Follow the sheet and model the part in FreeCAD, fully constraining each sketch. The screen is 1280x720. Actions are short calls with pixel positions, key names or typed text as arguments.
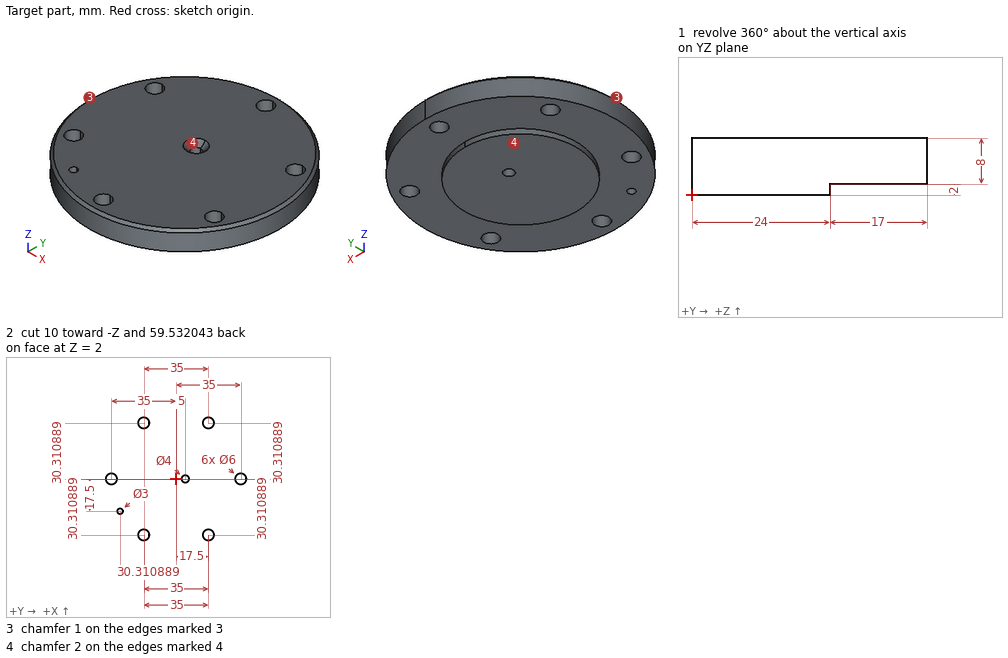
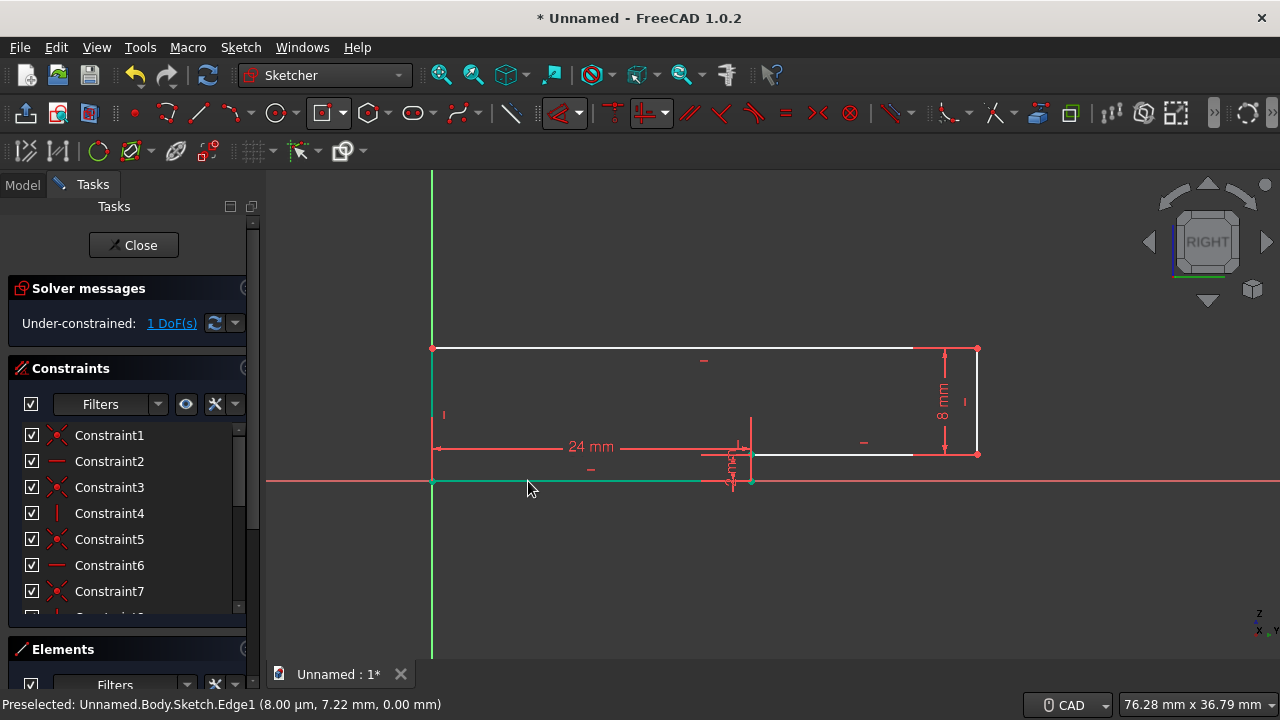
click(819, 455)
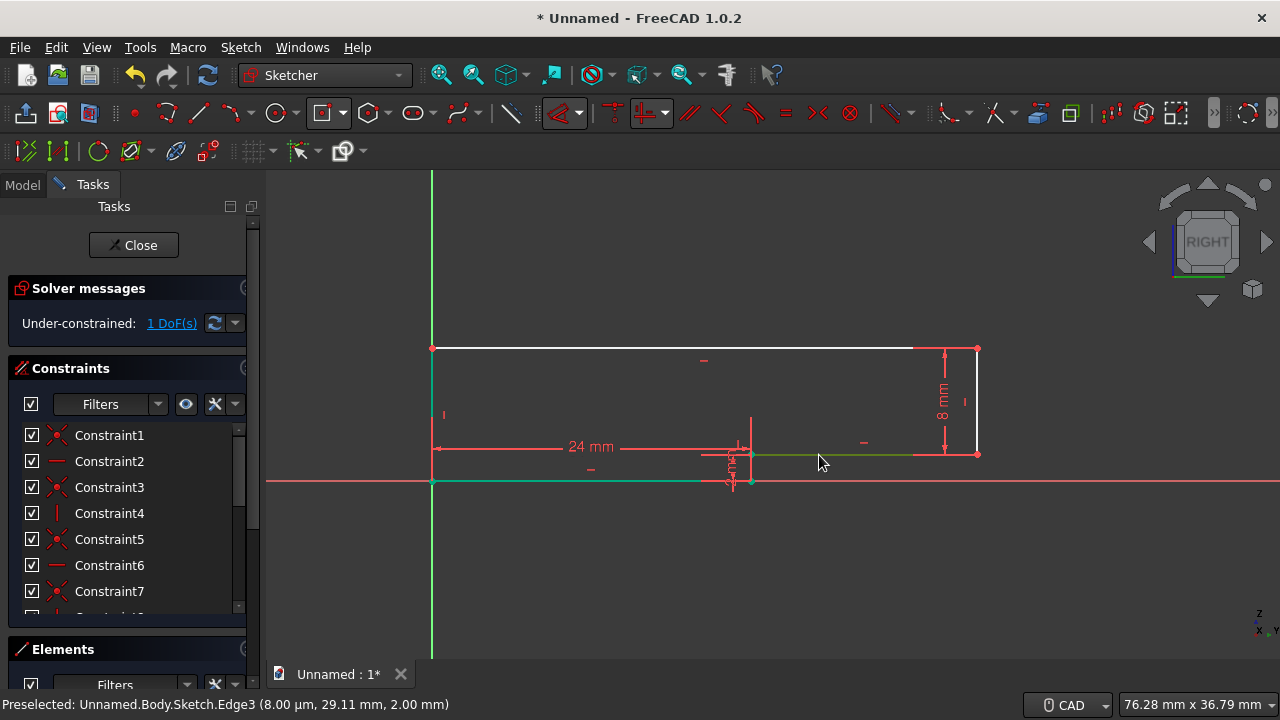
key(l)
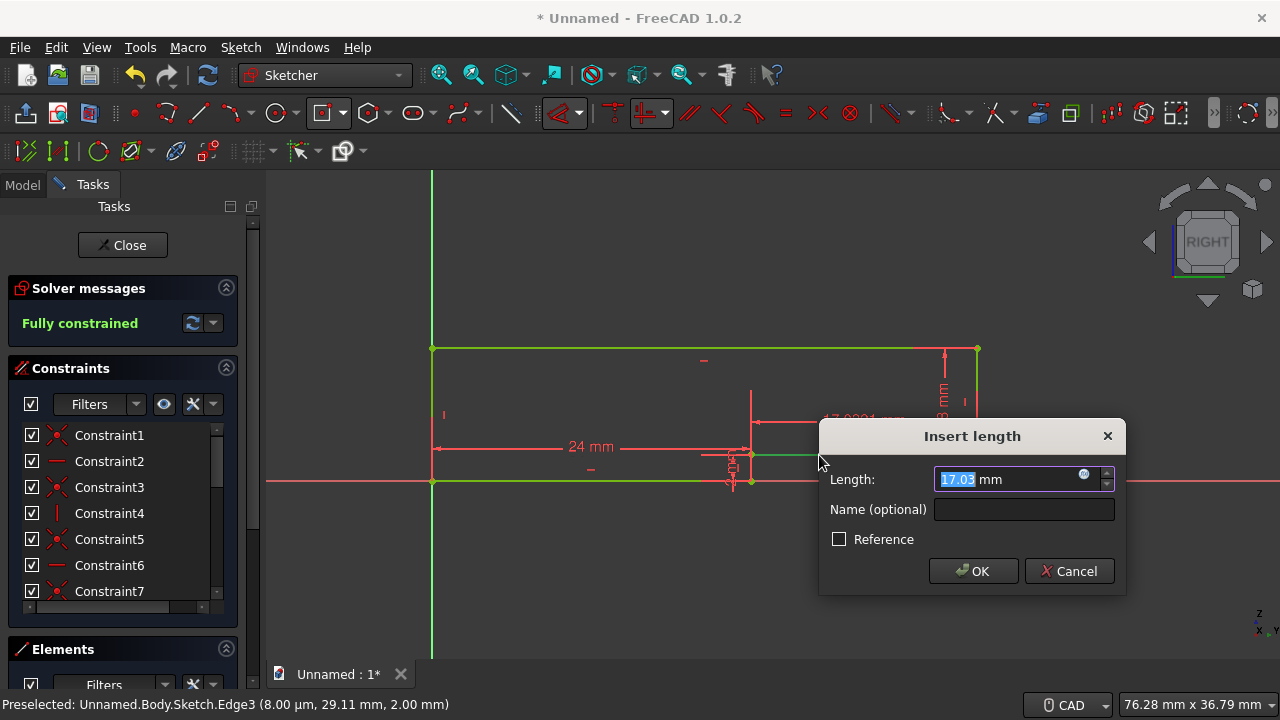
text(17)
key(Return)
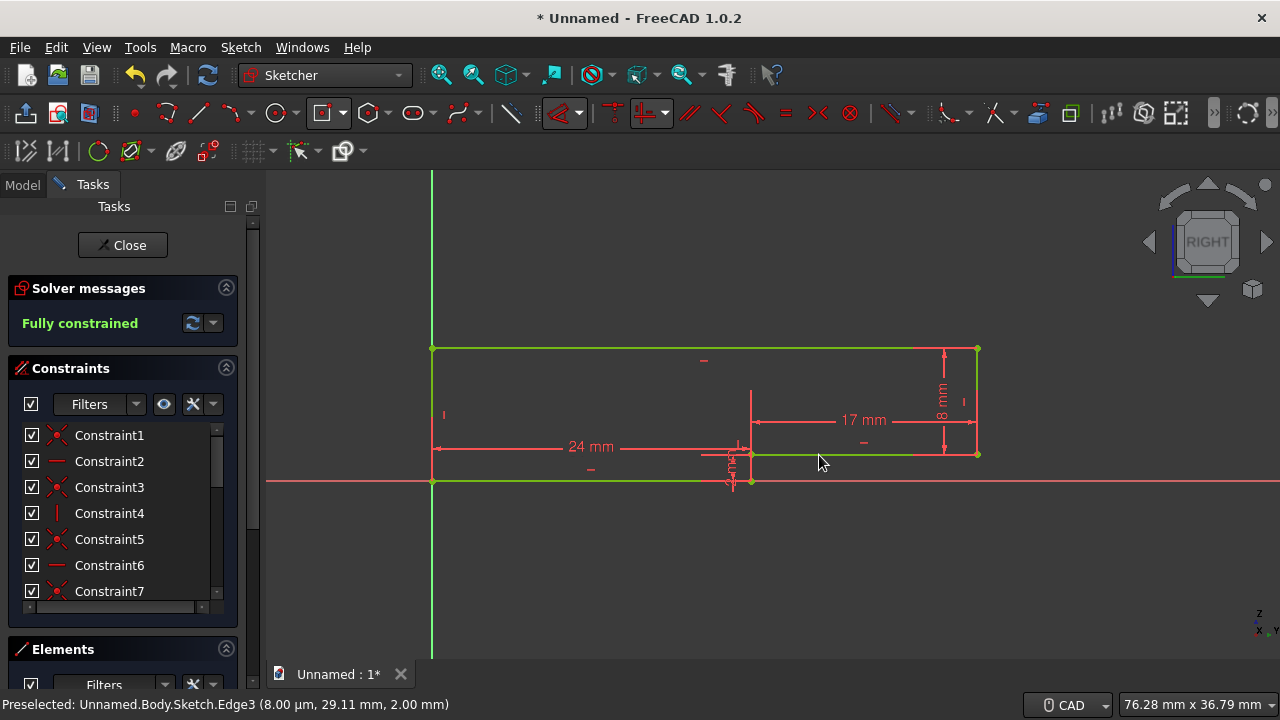
click(123, 245)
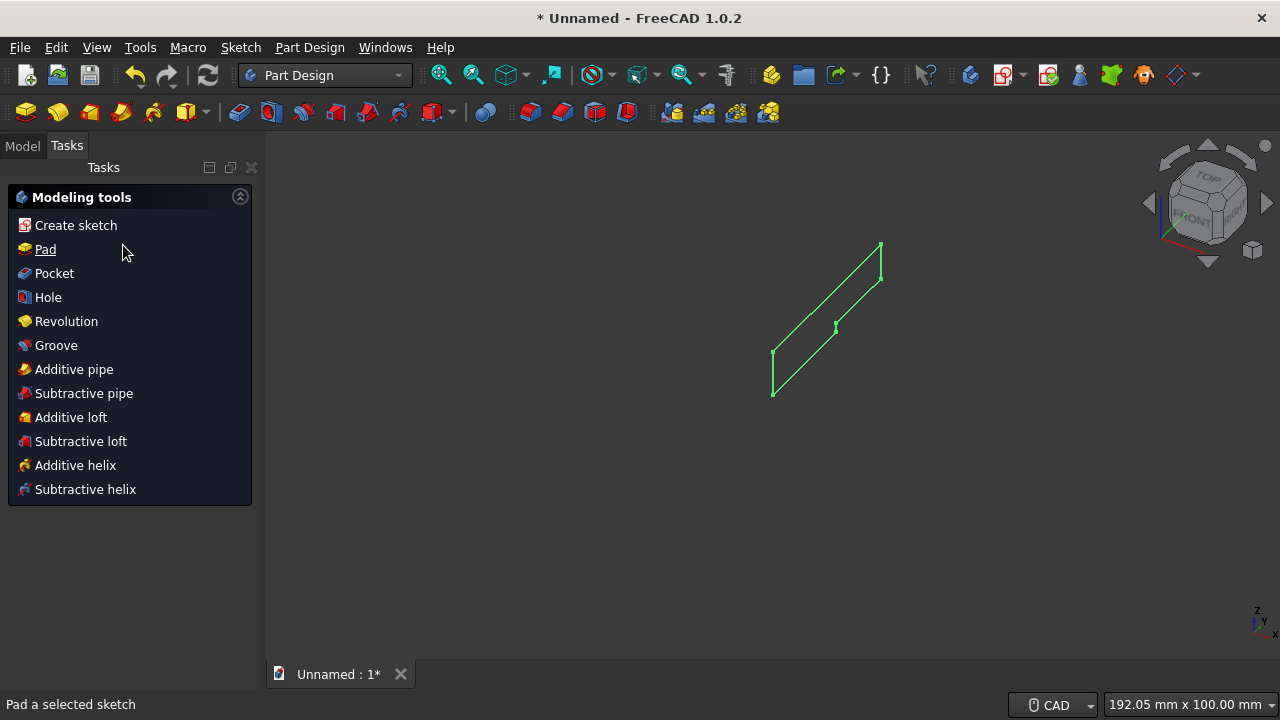
click(58, 112)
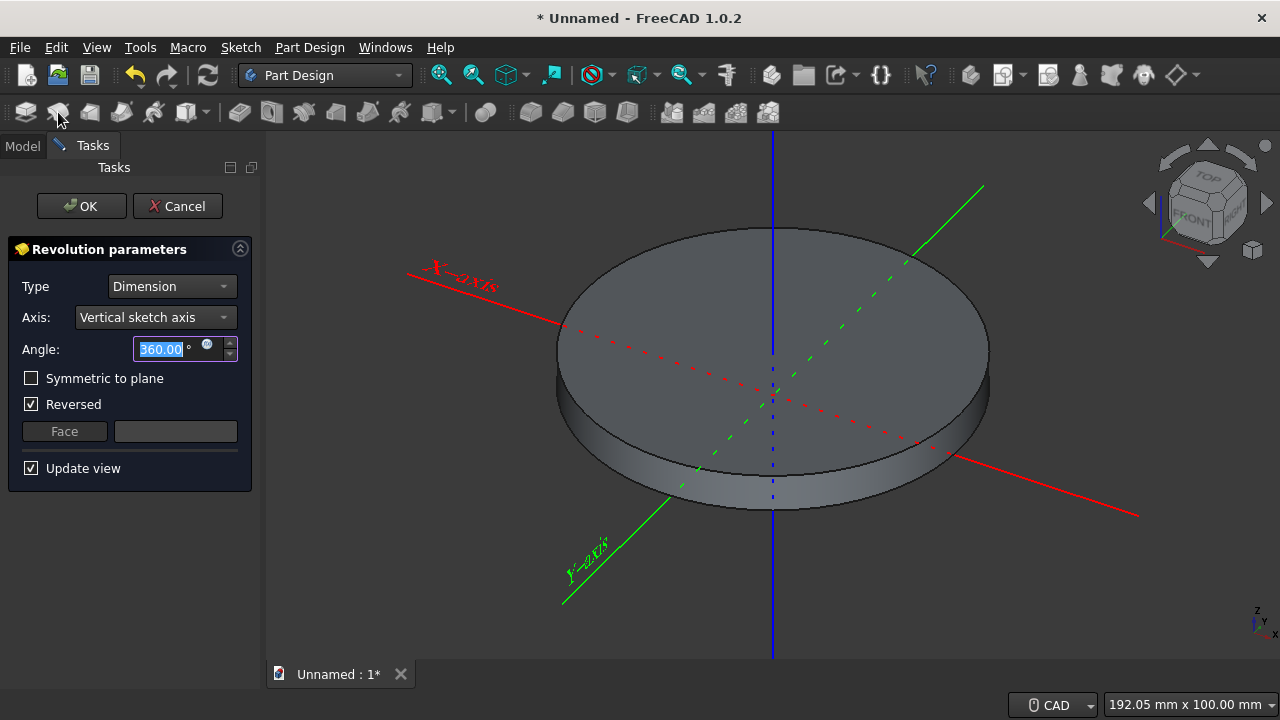
click(82, 206)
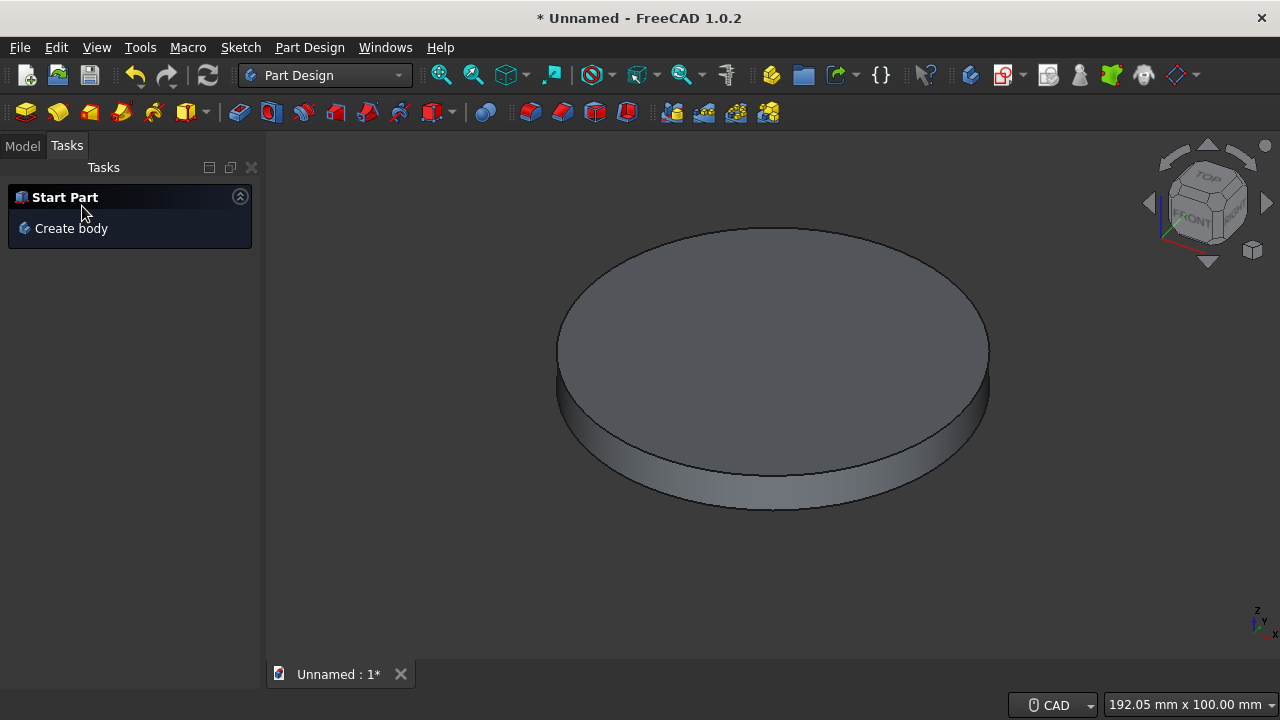
key(5)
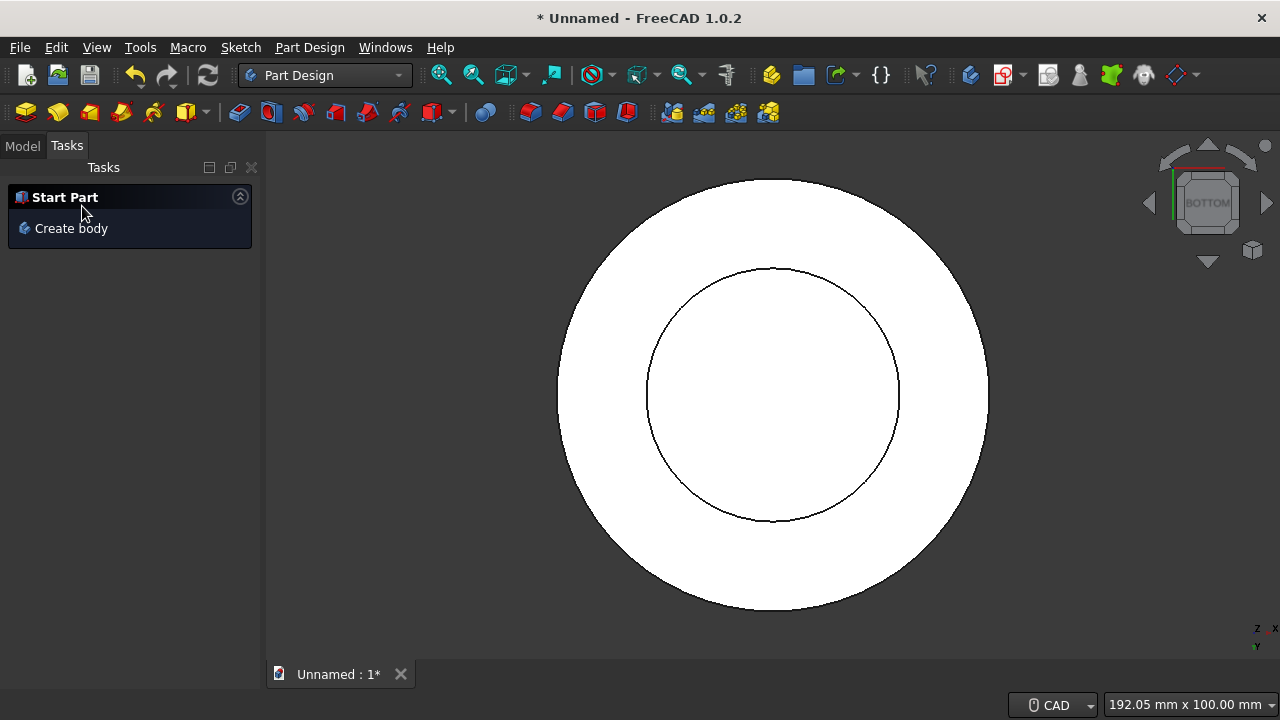
click(897, 270)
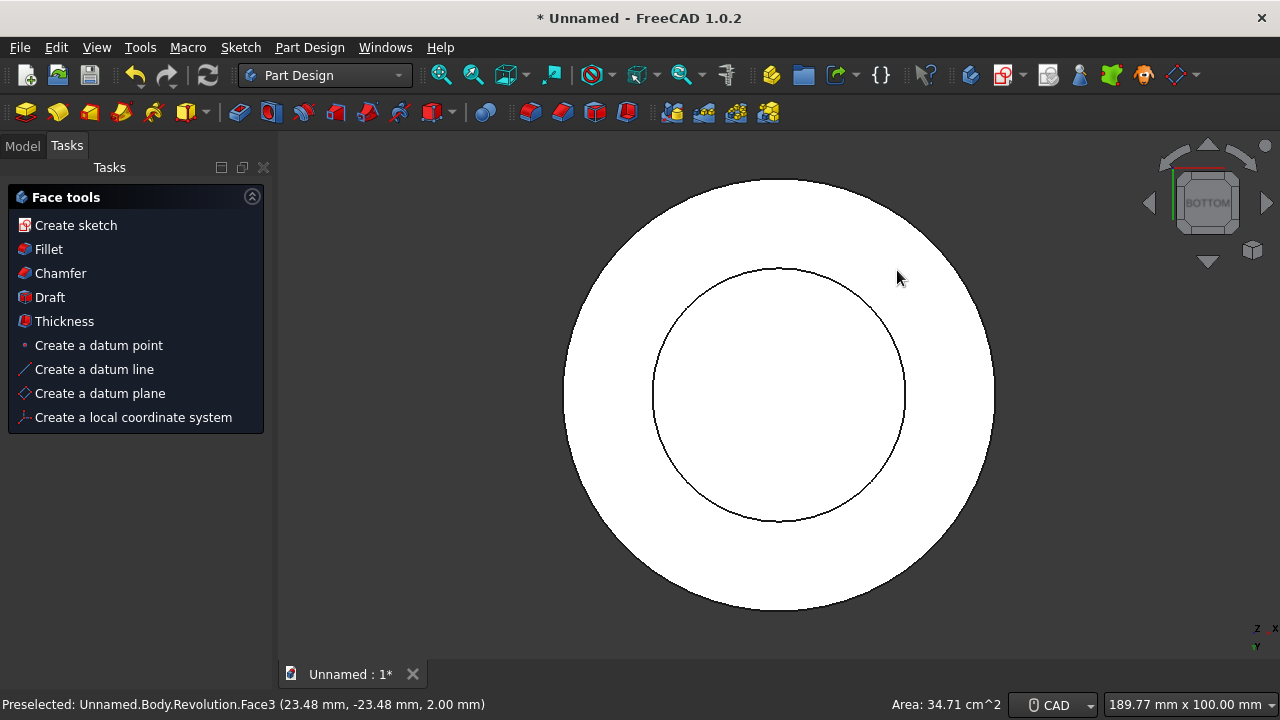
click(1004, 76)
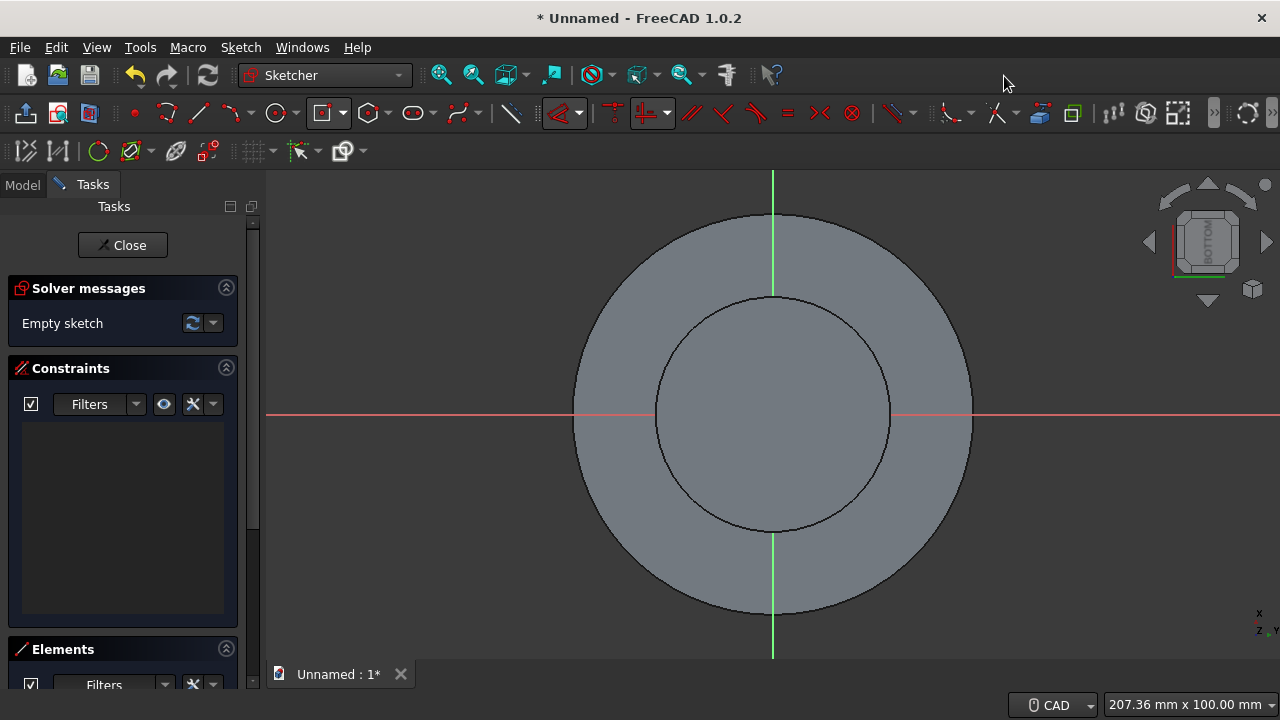
click(90, 114)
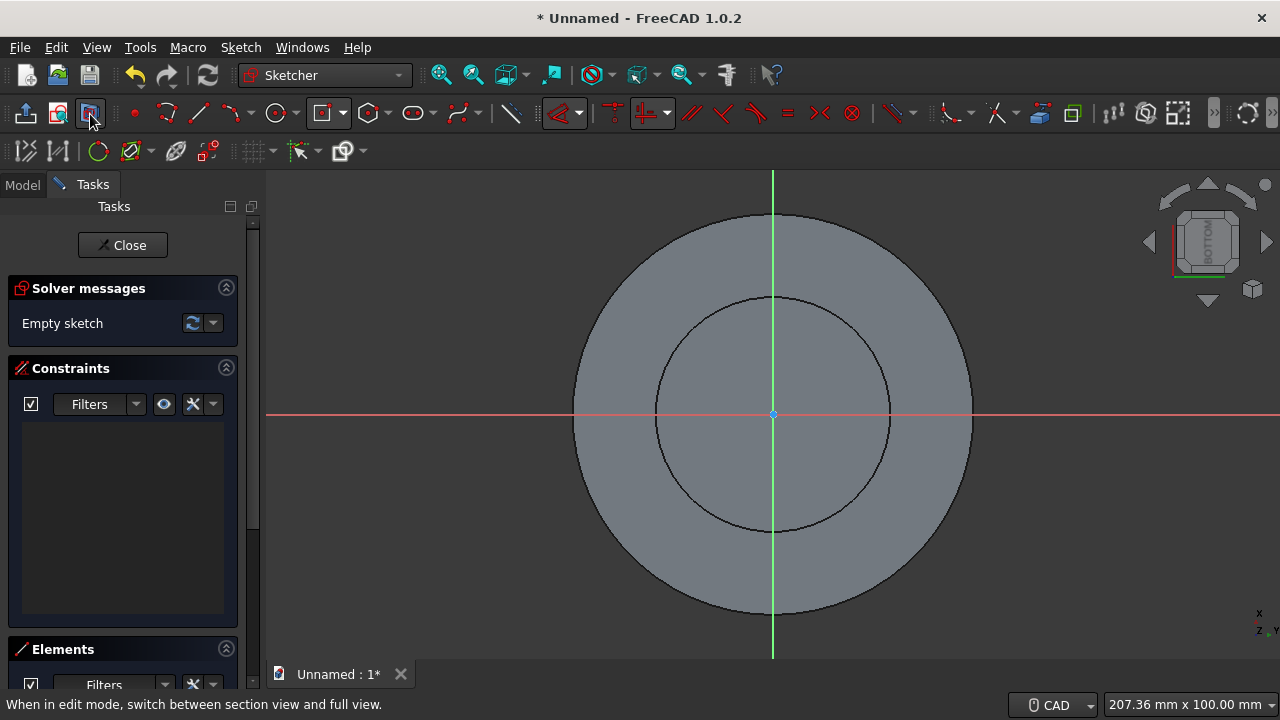
click(276, 114)